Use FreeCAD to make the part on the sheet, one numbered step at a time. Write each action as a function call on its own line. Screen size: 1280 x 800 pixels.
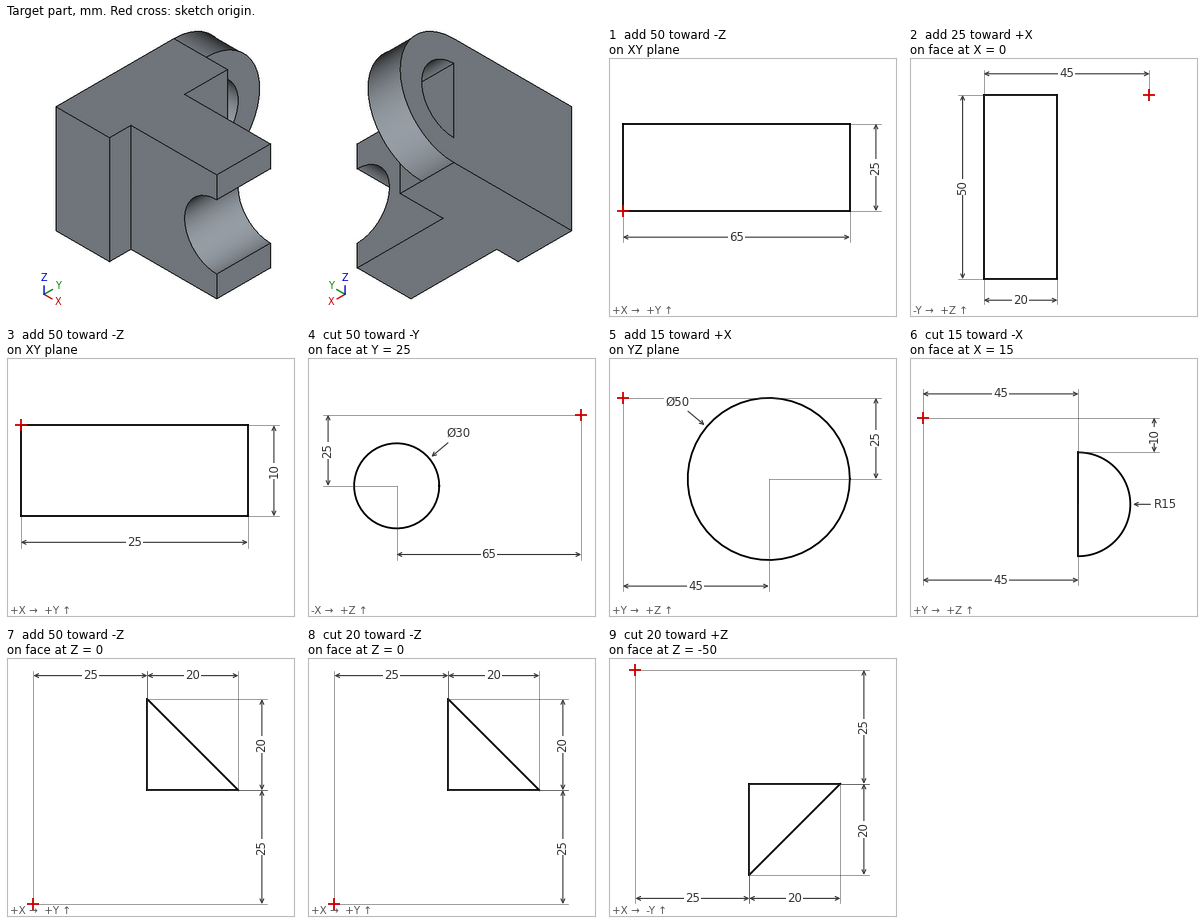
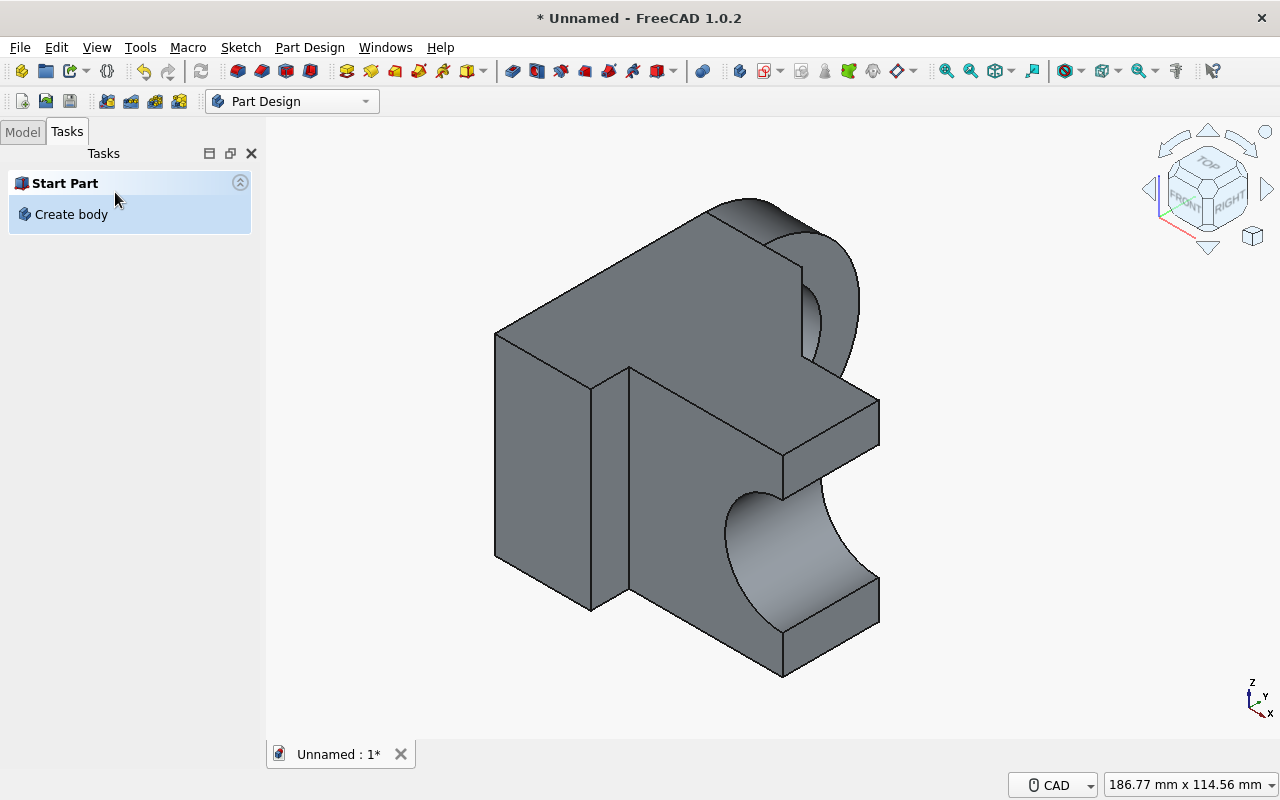
click(689, 323)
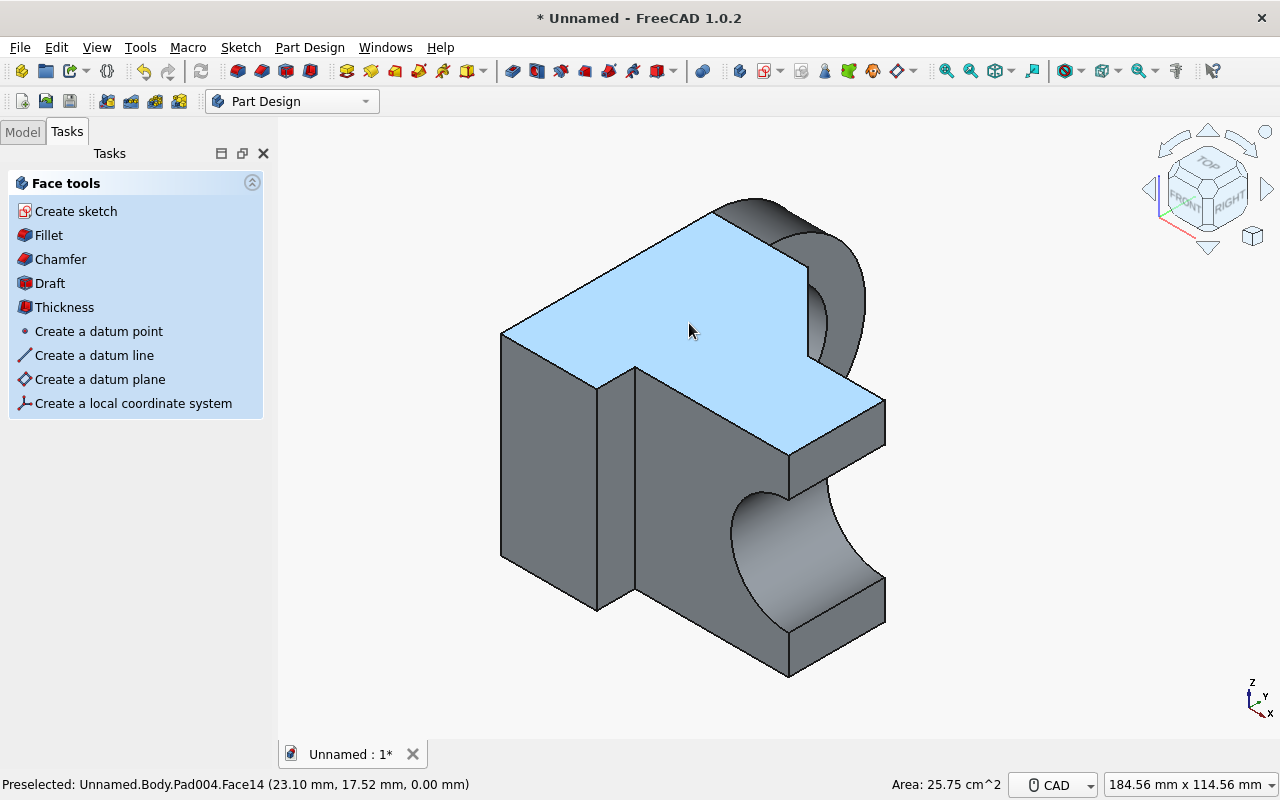
click(764, 72)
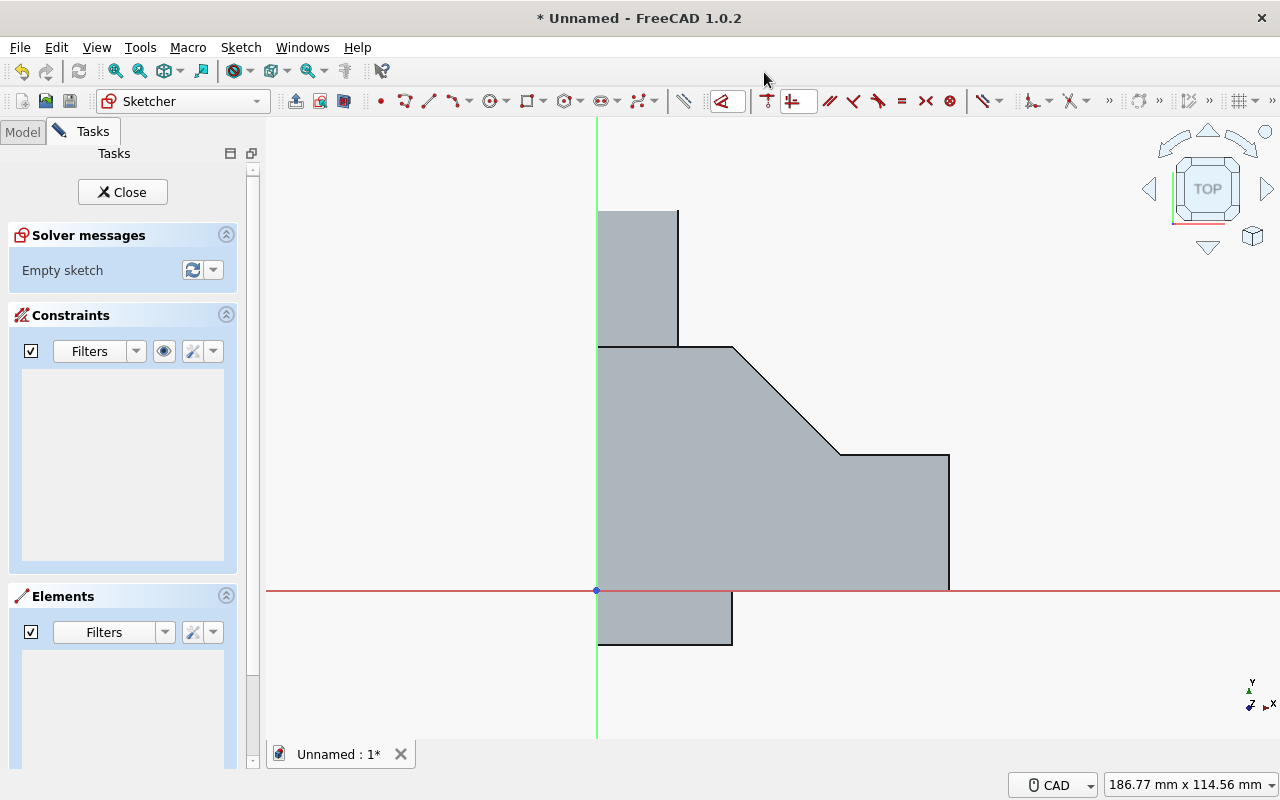
scroll(748, 552, up, 2)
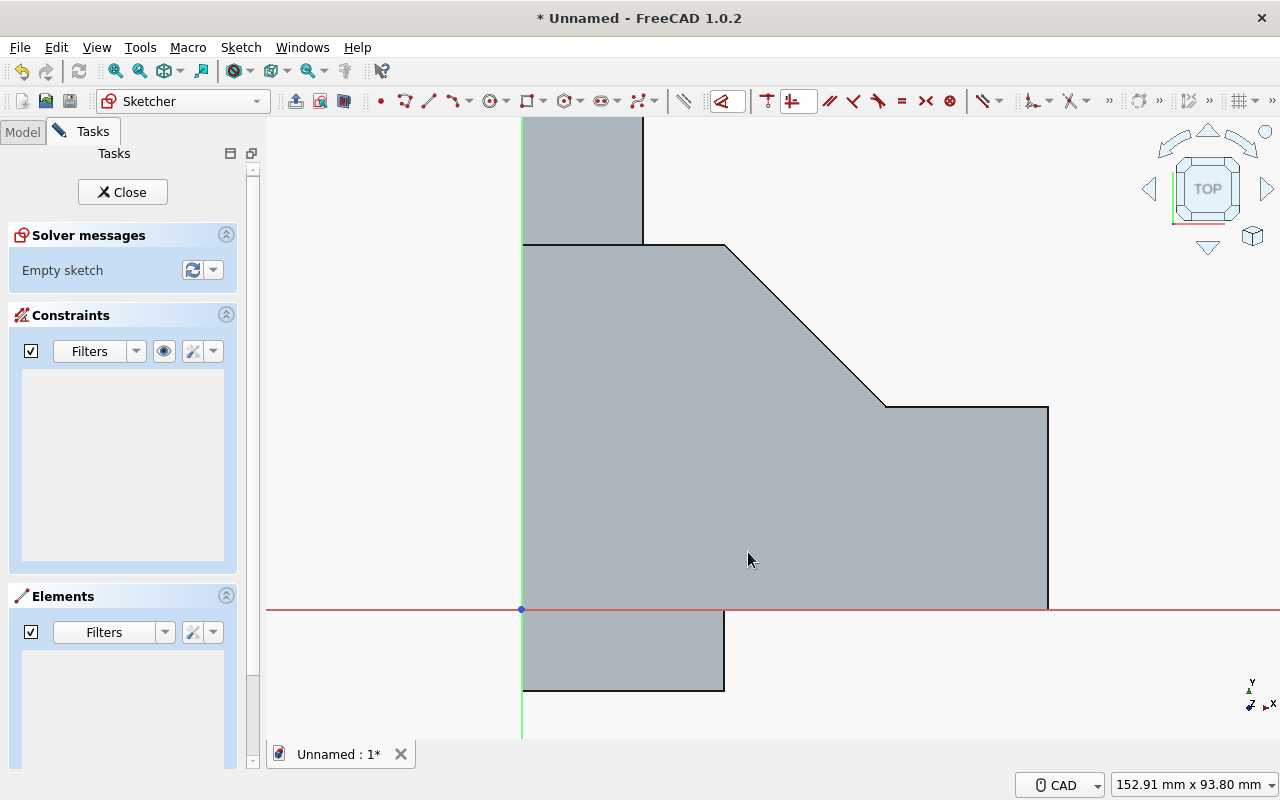
click(406, 102)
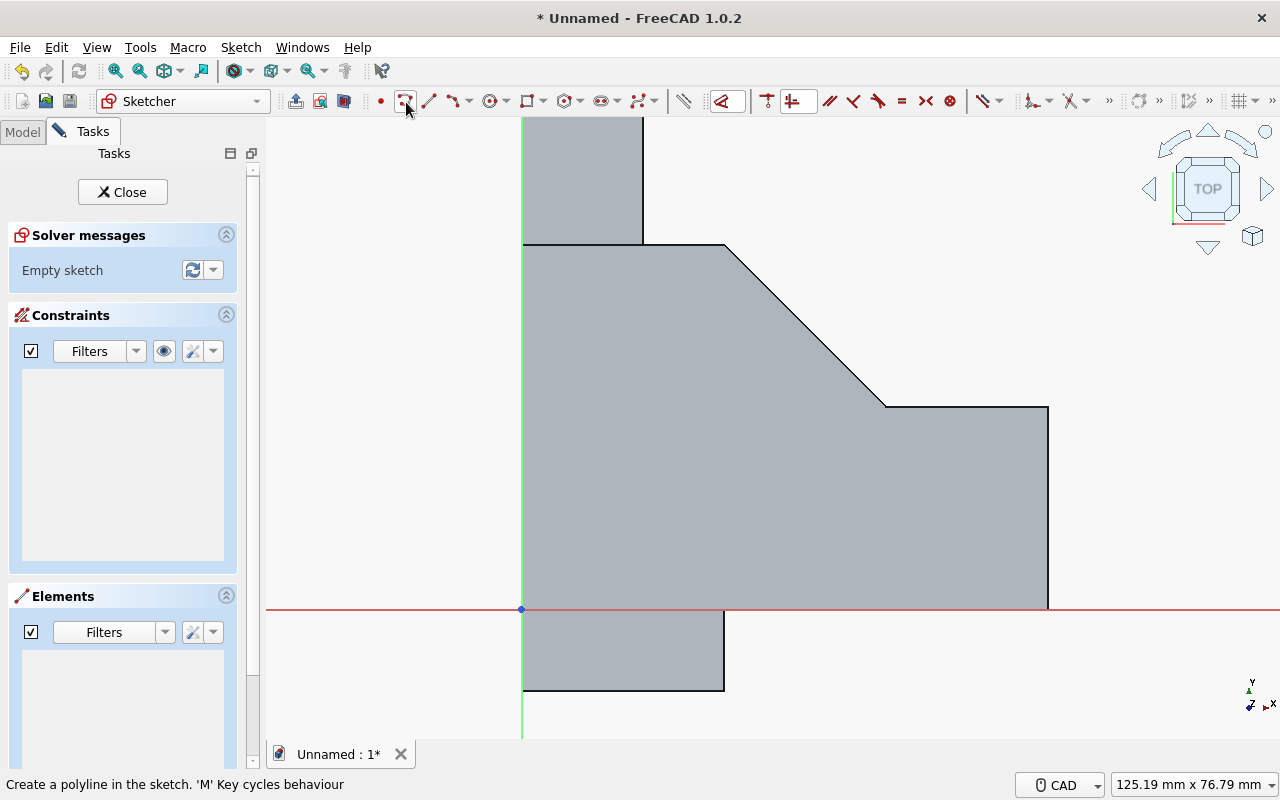
click(724, 407)
click(886, 407)
click(724, 245)
click(724, 408)
key(Escape)
key(Escape)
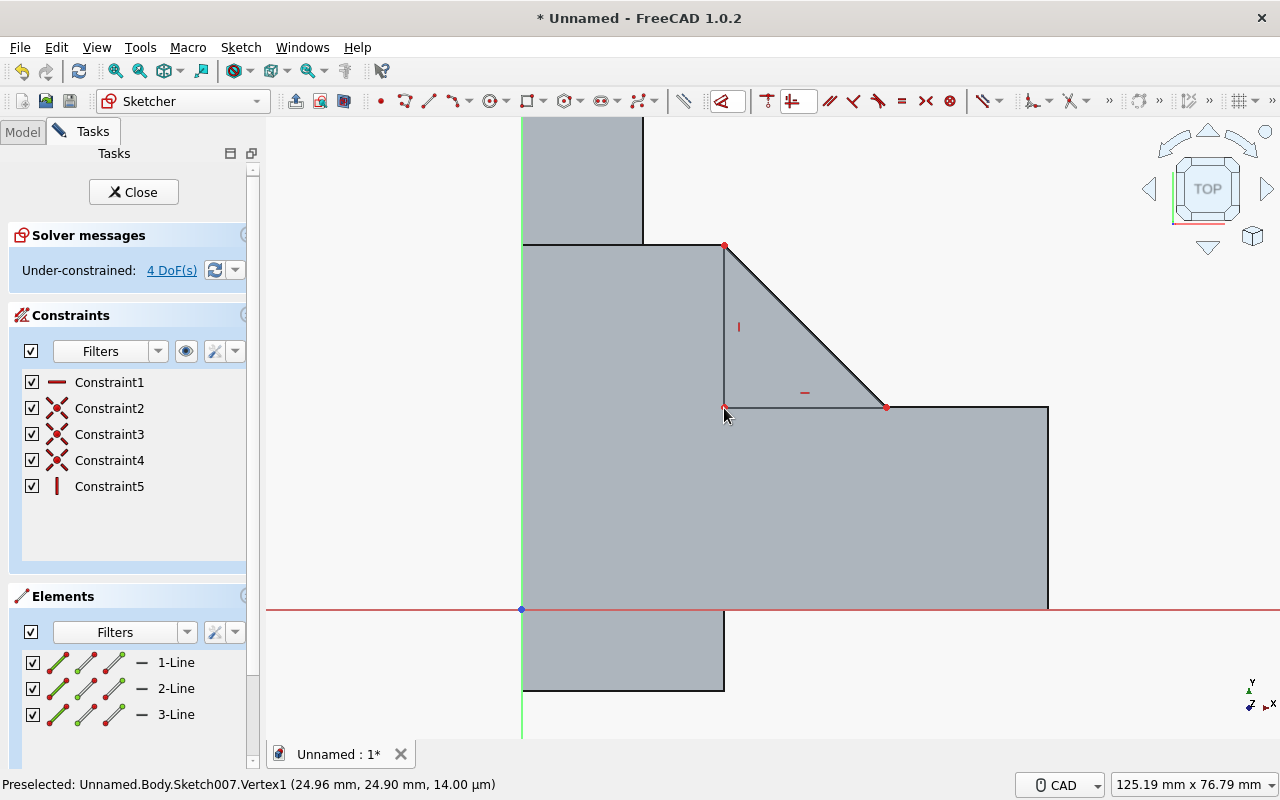
click(773, 408)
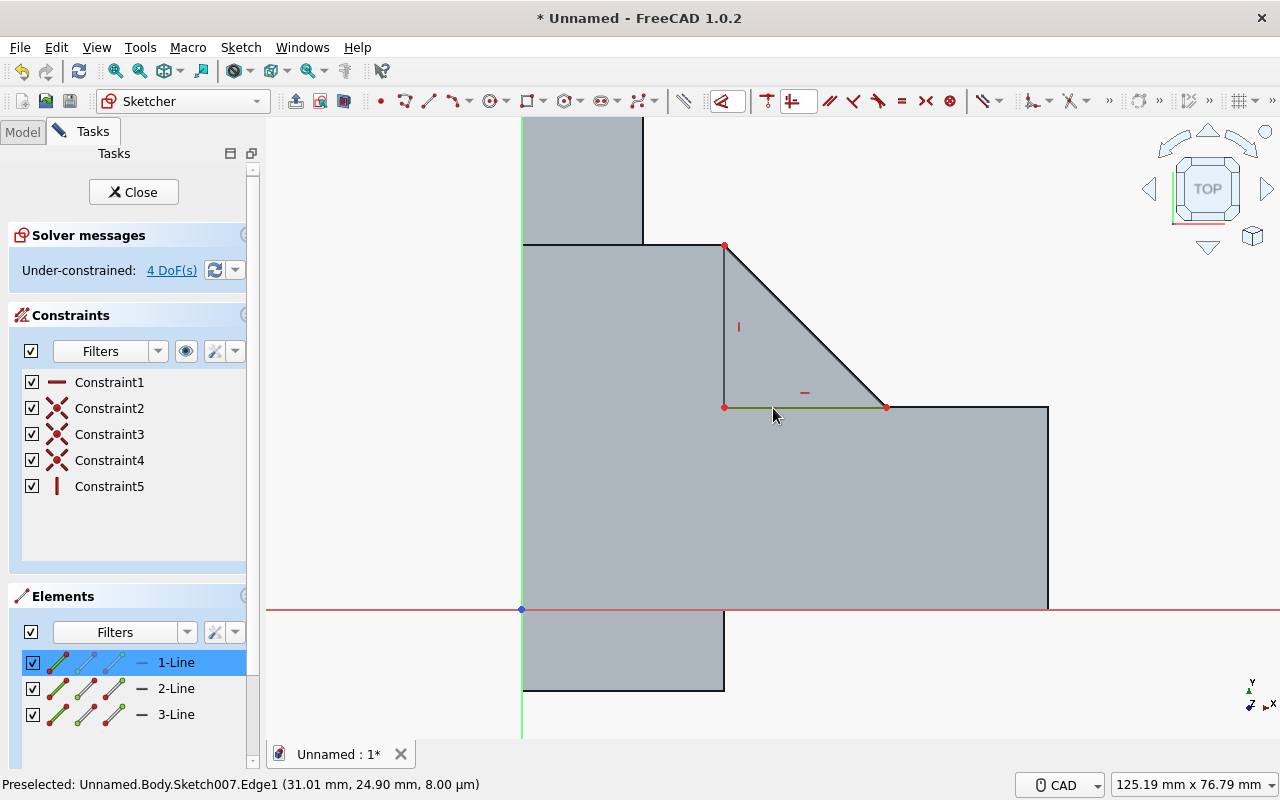
key(l)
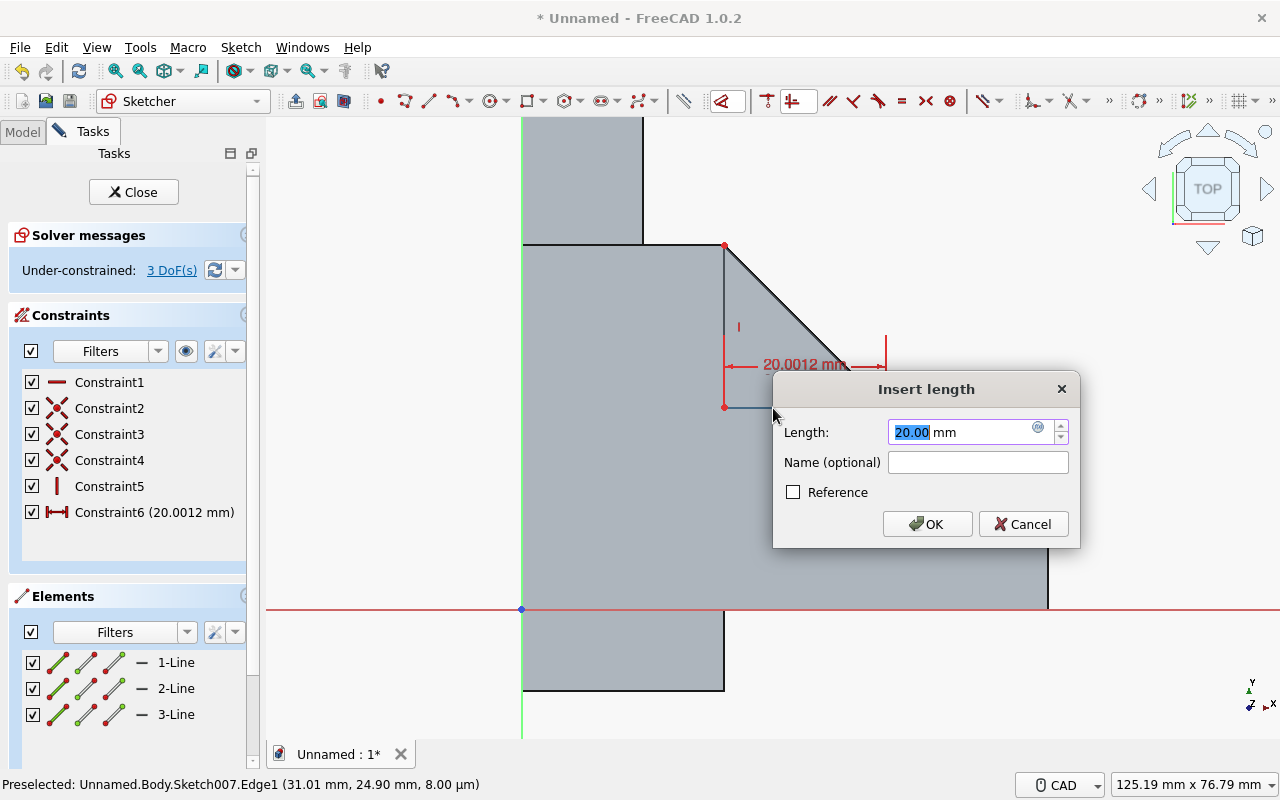
text(20)
key(Return)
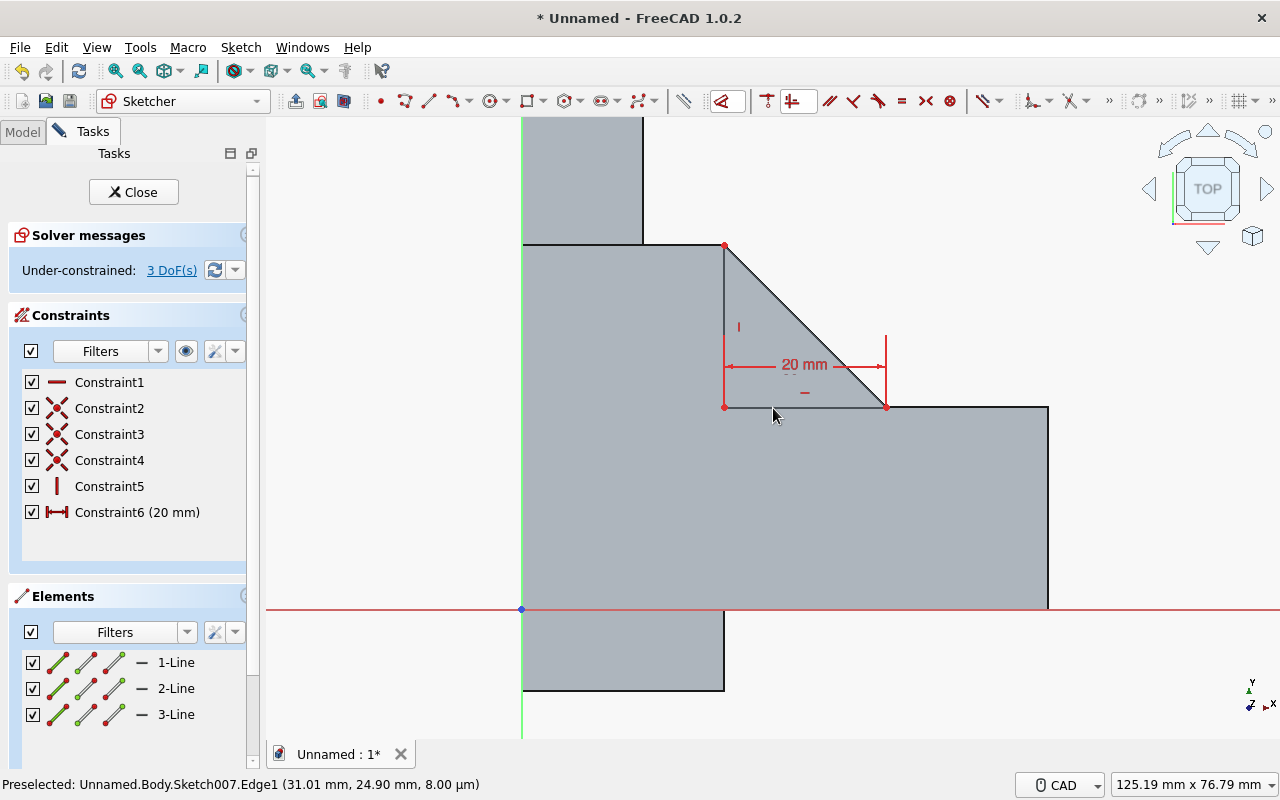
click(724, 295)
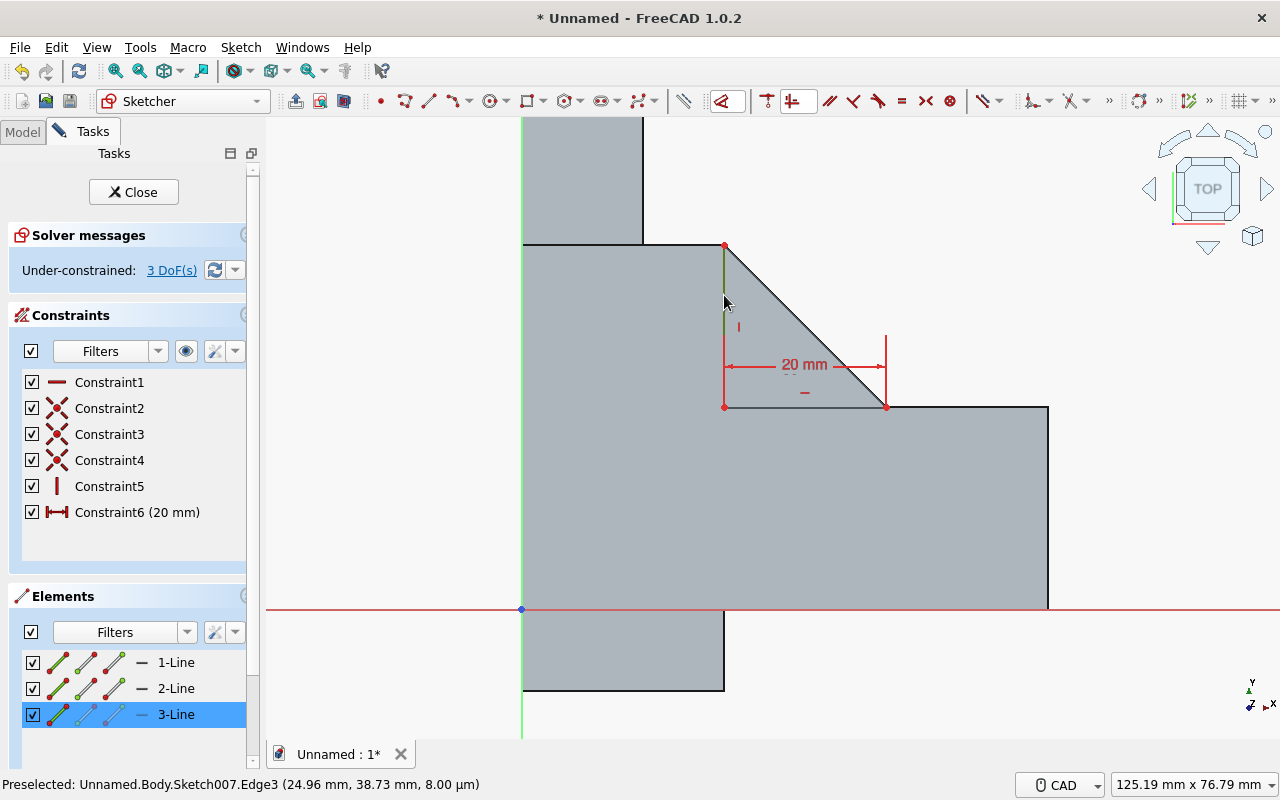
click(740, 102)